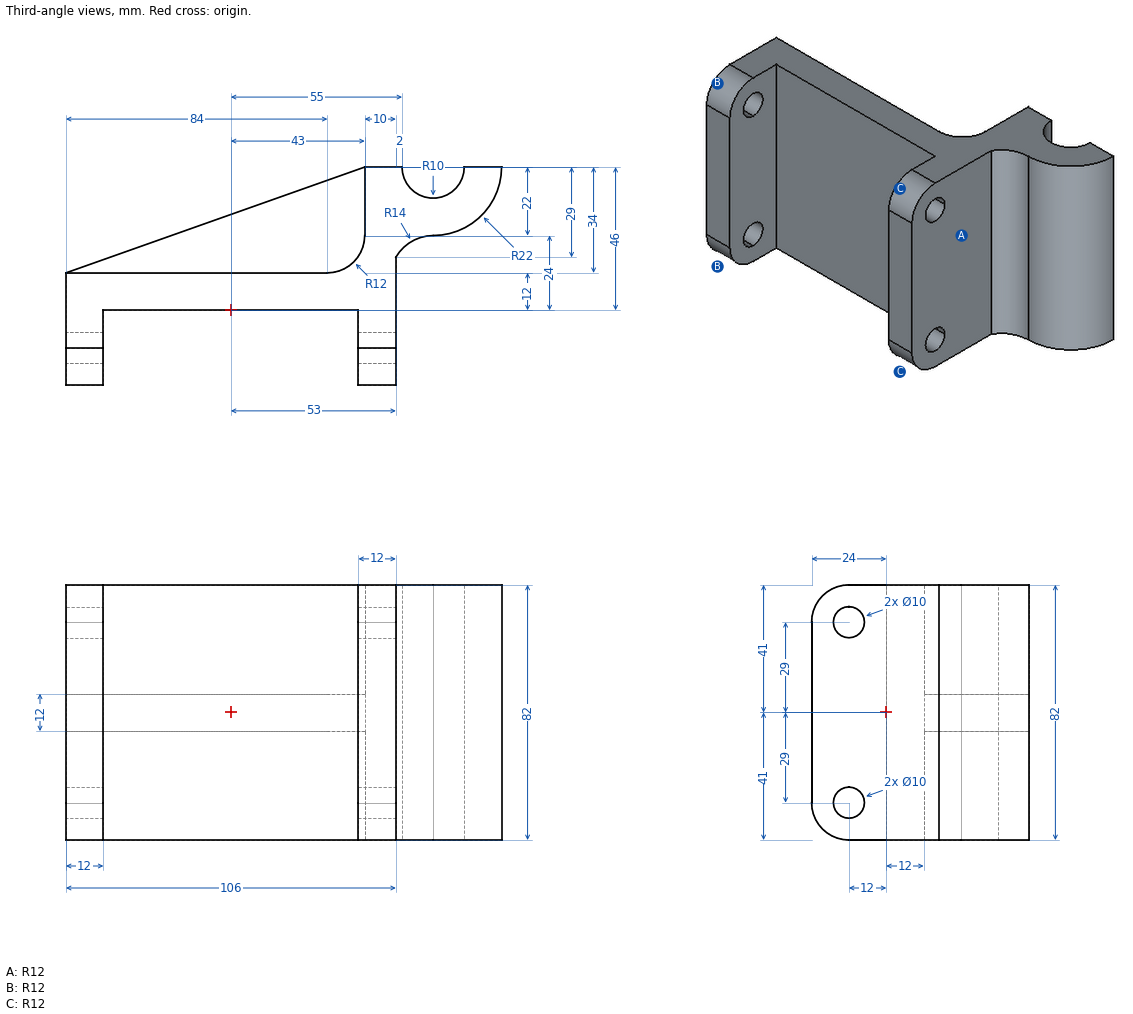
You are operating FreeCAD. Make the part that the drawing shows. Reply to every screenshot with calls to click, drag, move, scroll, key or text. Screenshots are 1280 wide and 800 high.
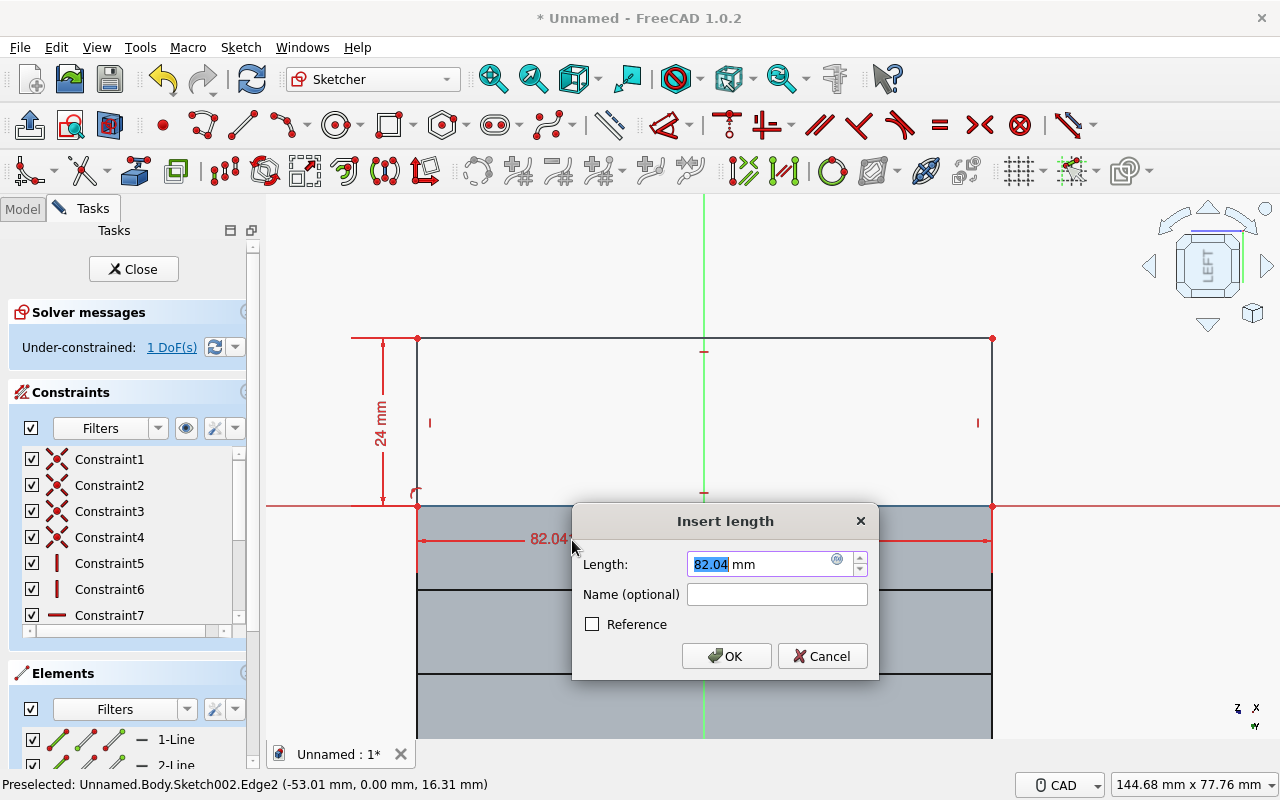
text(82)
key(Return)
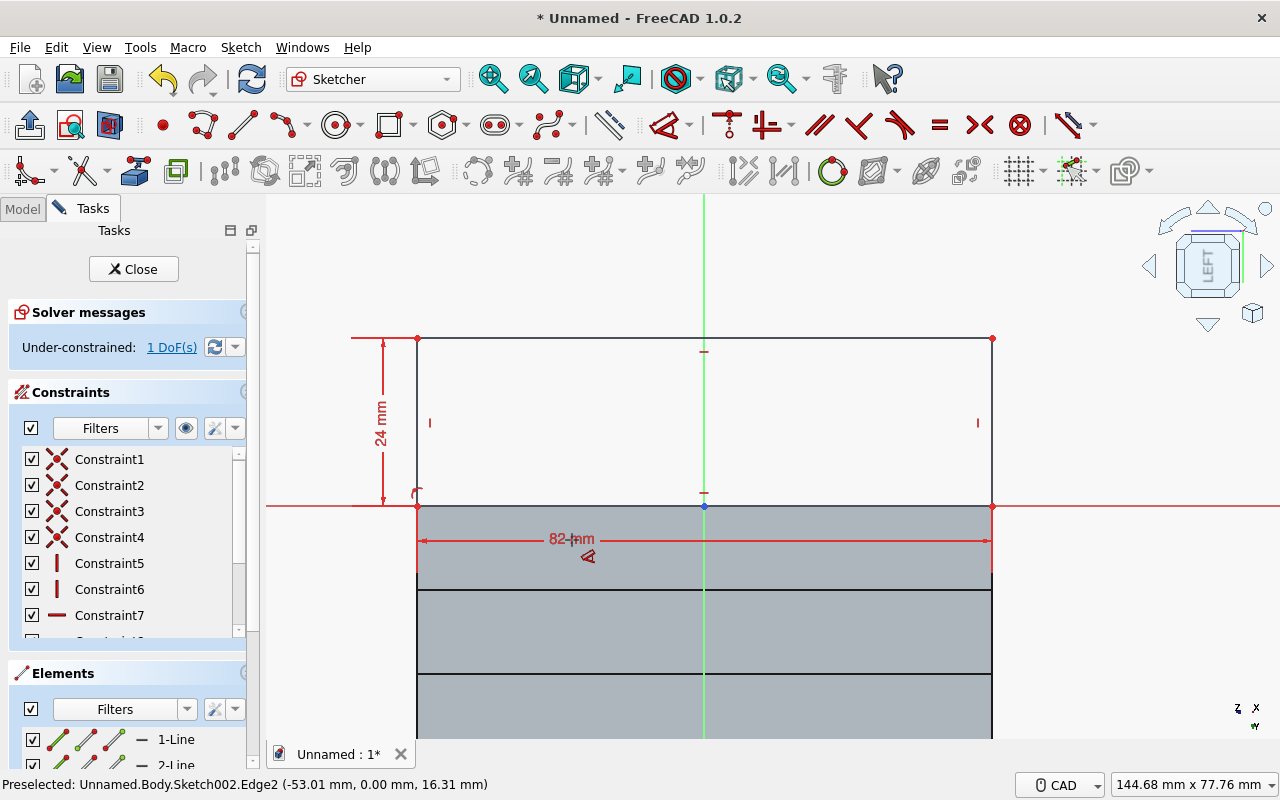
click(417, 338)
click(495, 540)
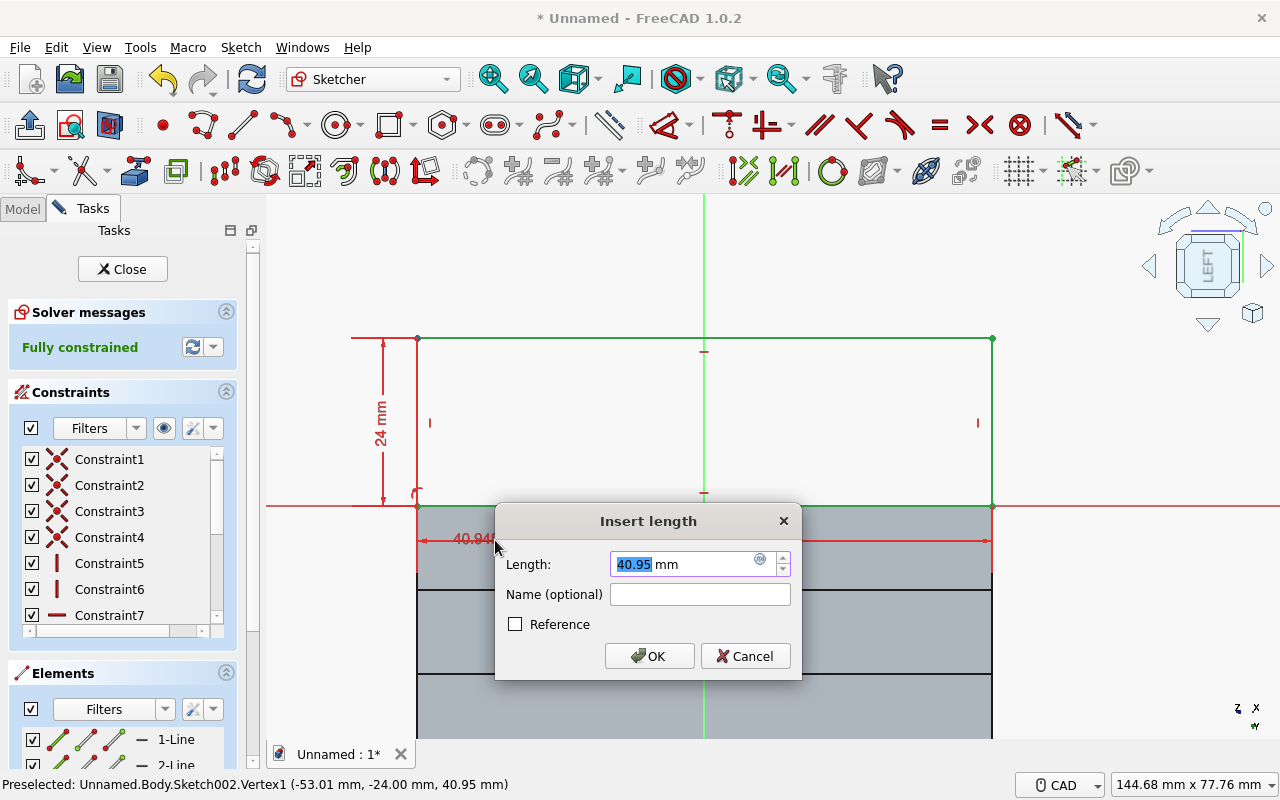
text(41)
key(Return)
key(Escape)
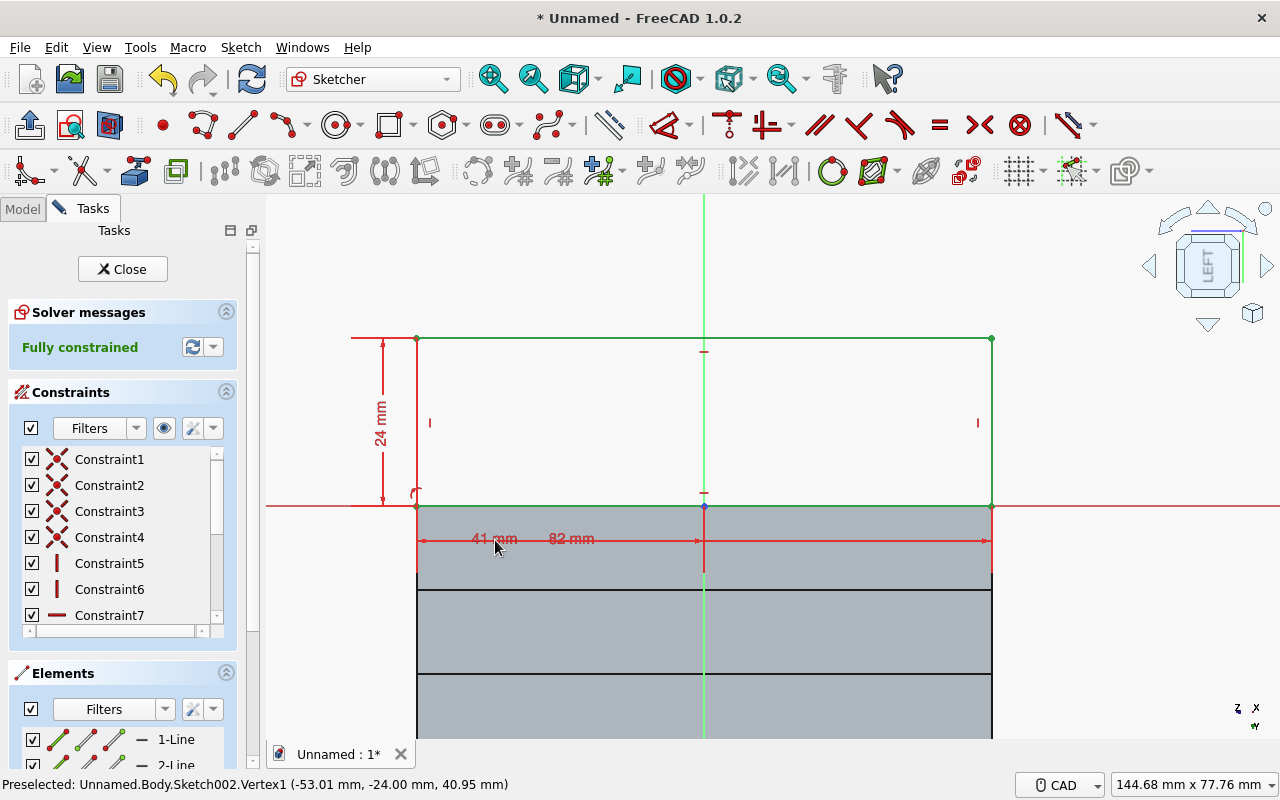
click(123, 269)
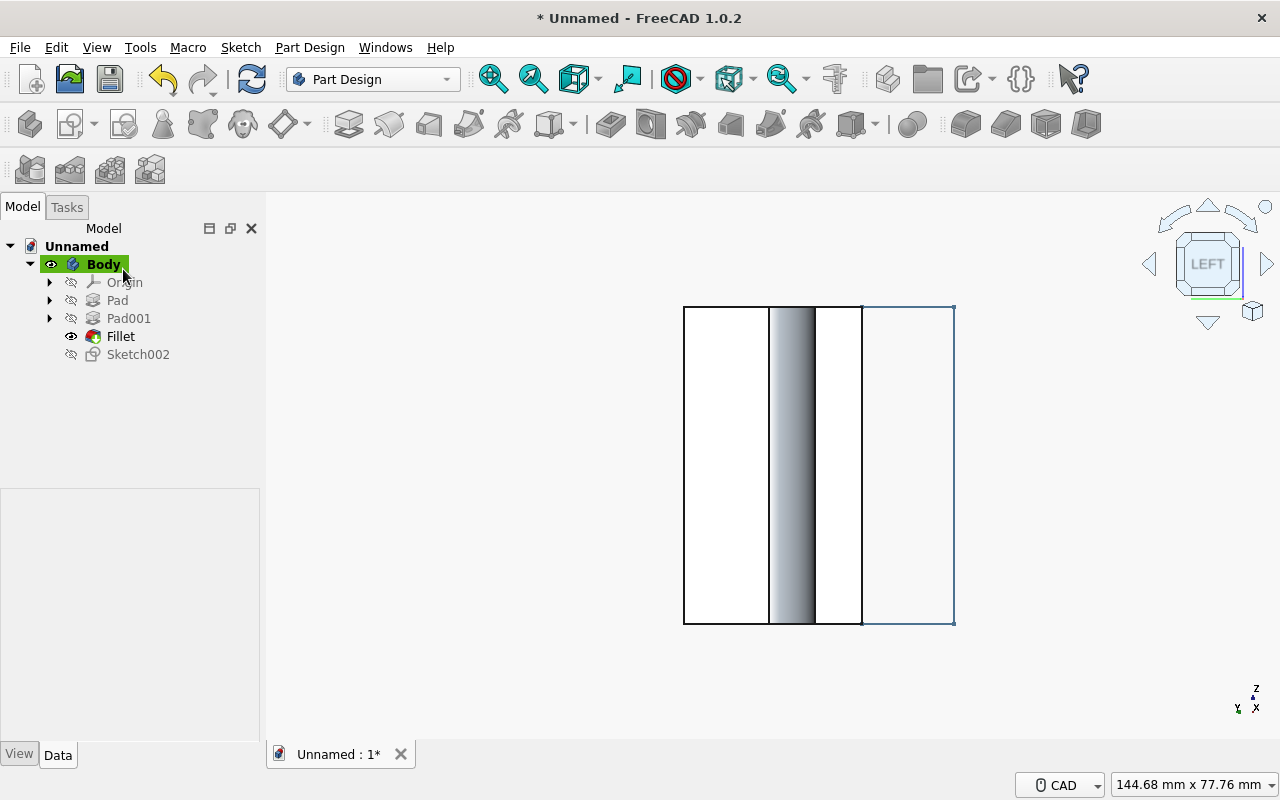
click(350, 124)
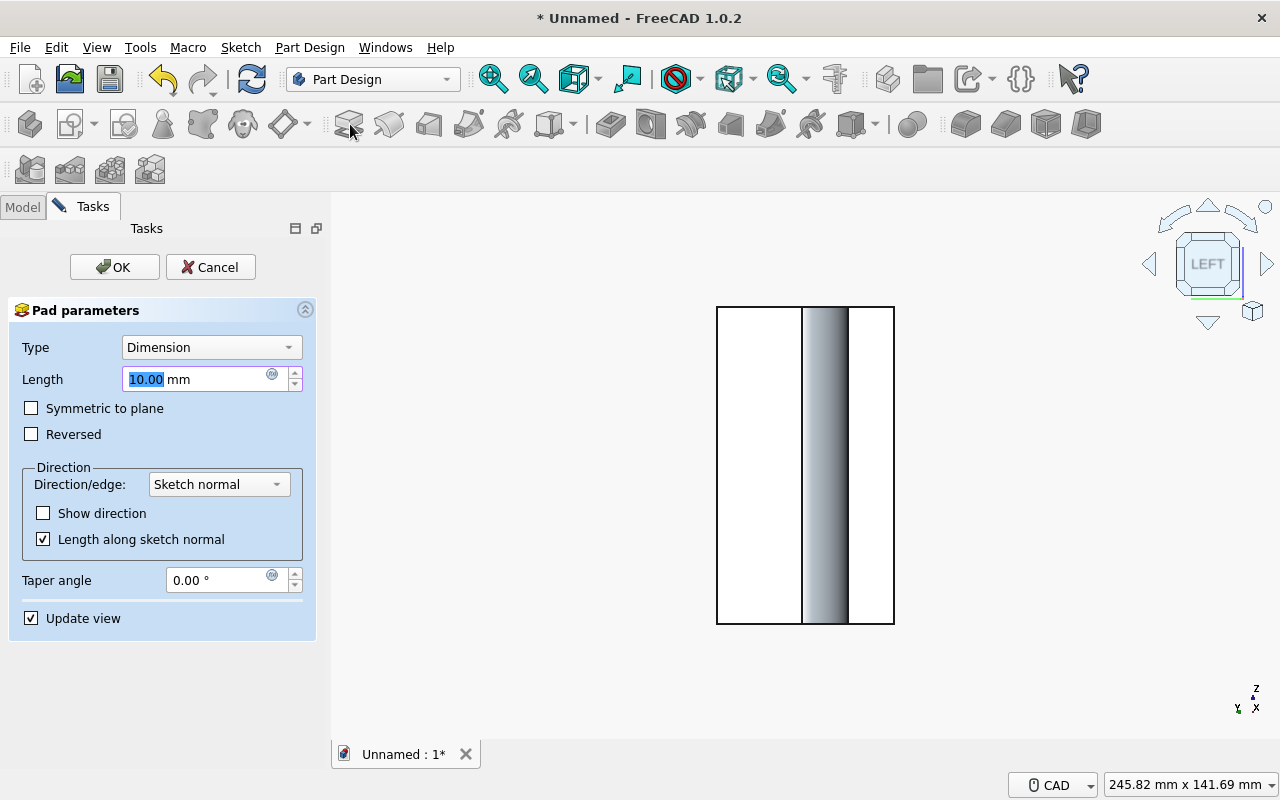
text(12)
key(Tab)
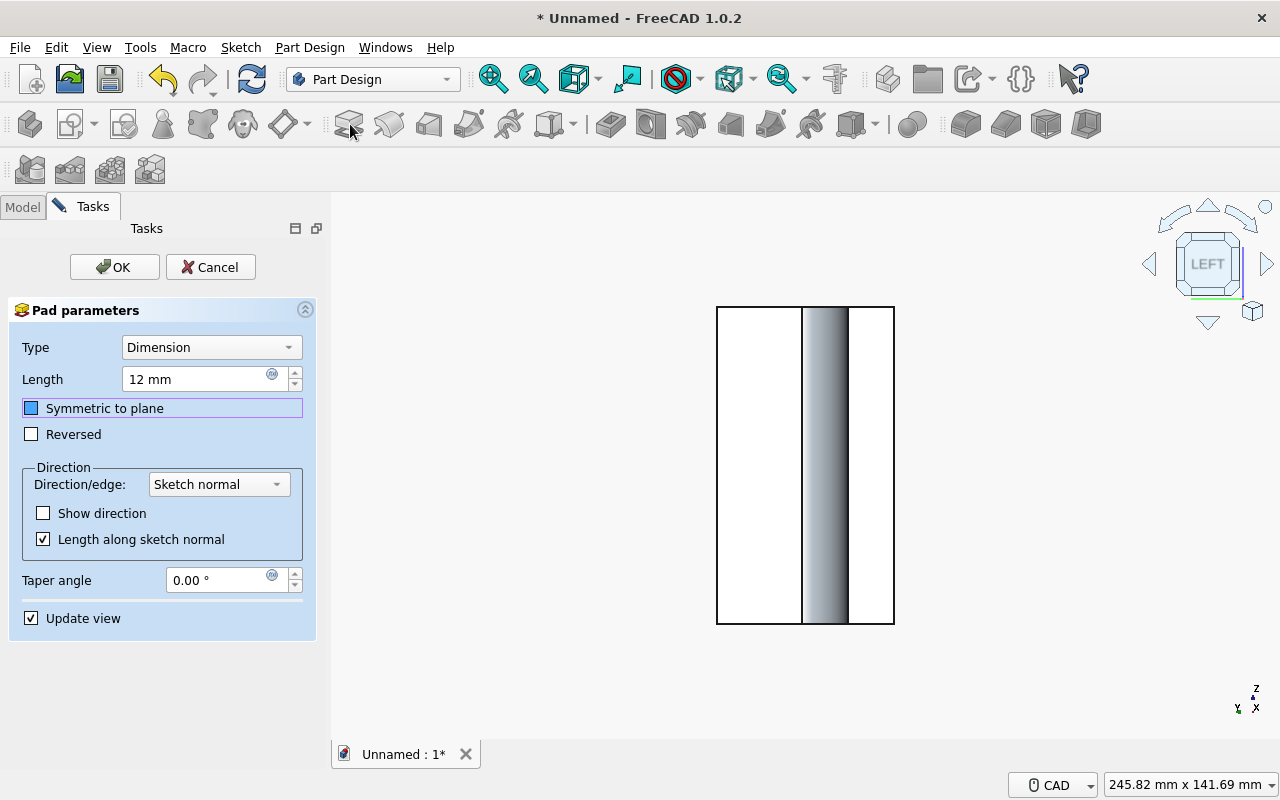
click(30, 434)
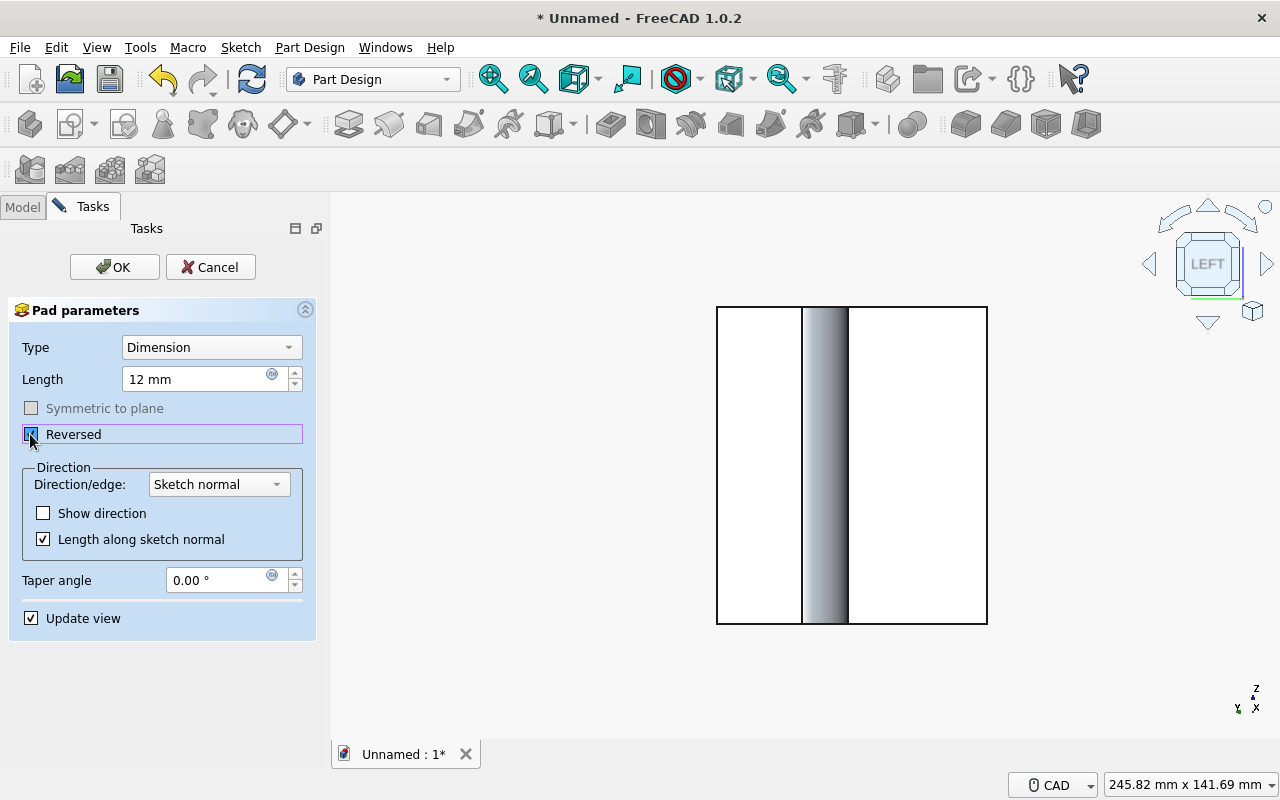
click(115, 267)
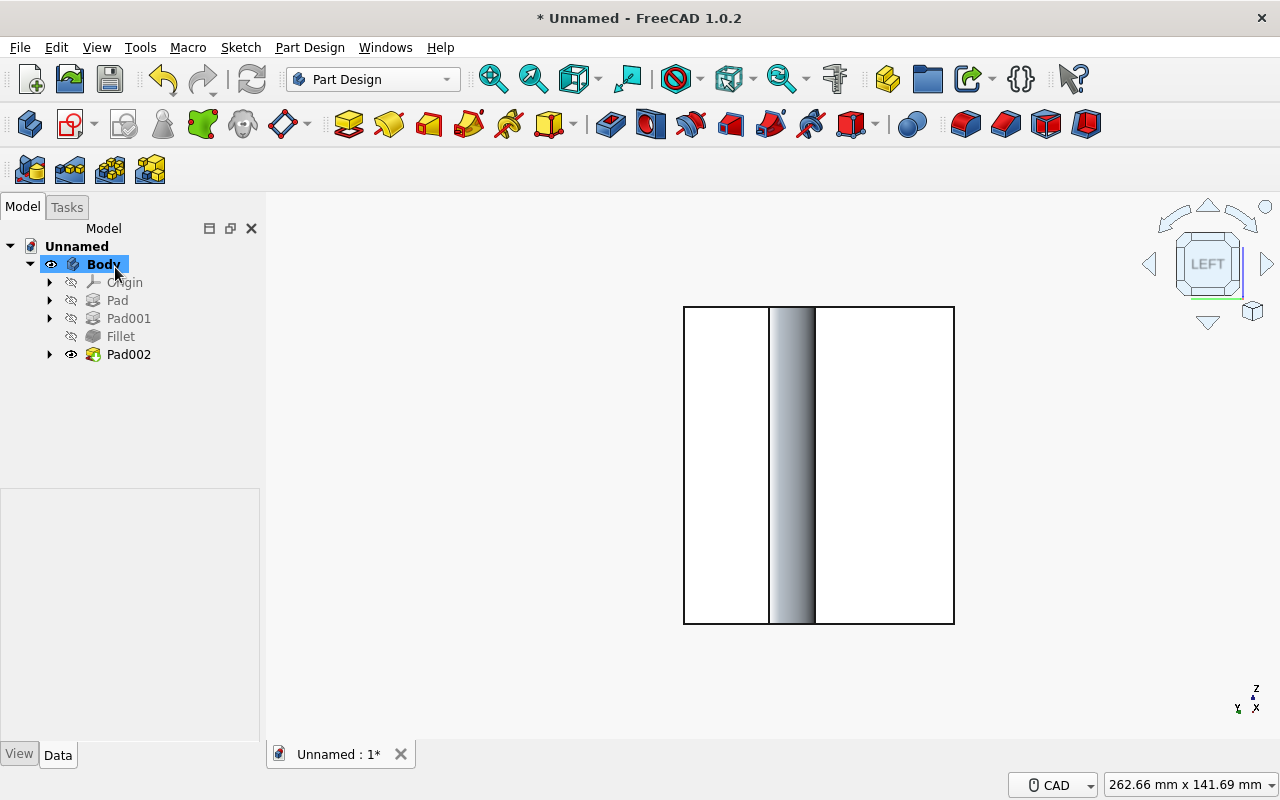
key(0)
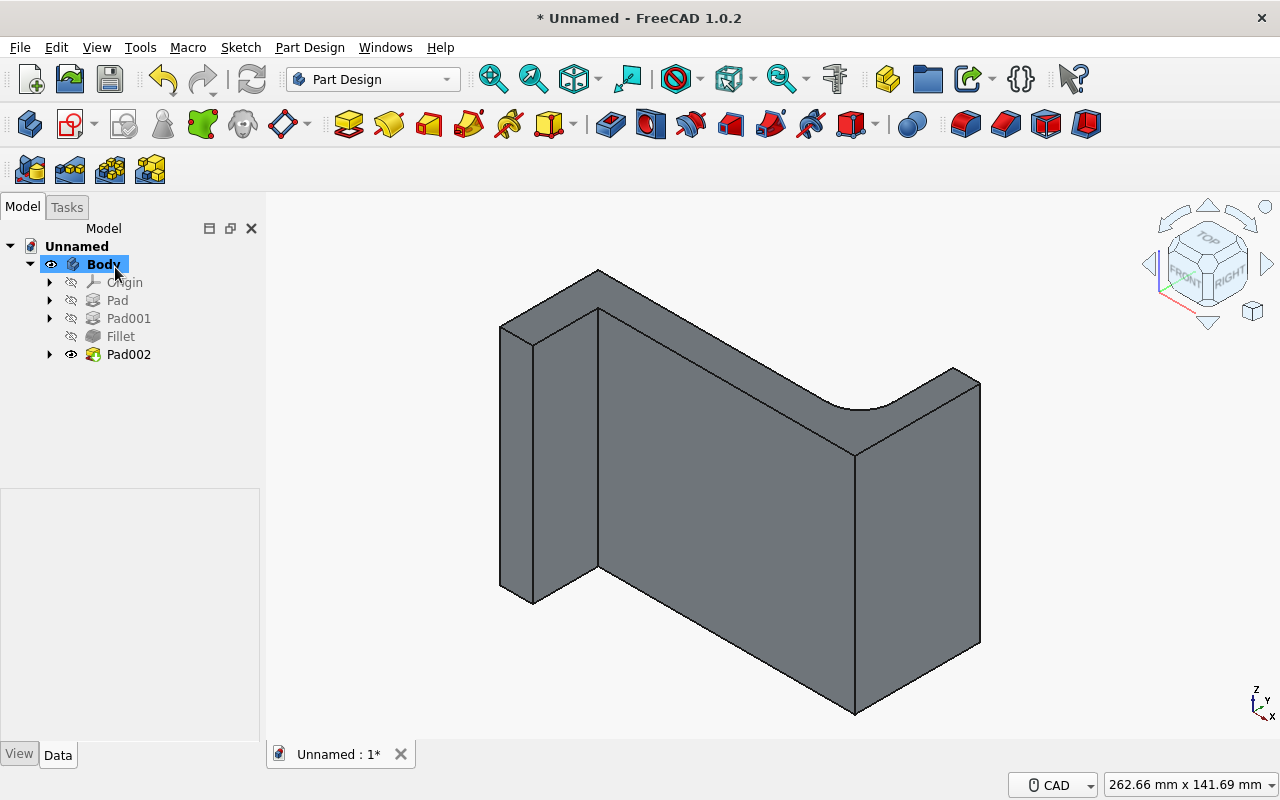
key(v)
key(f)